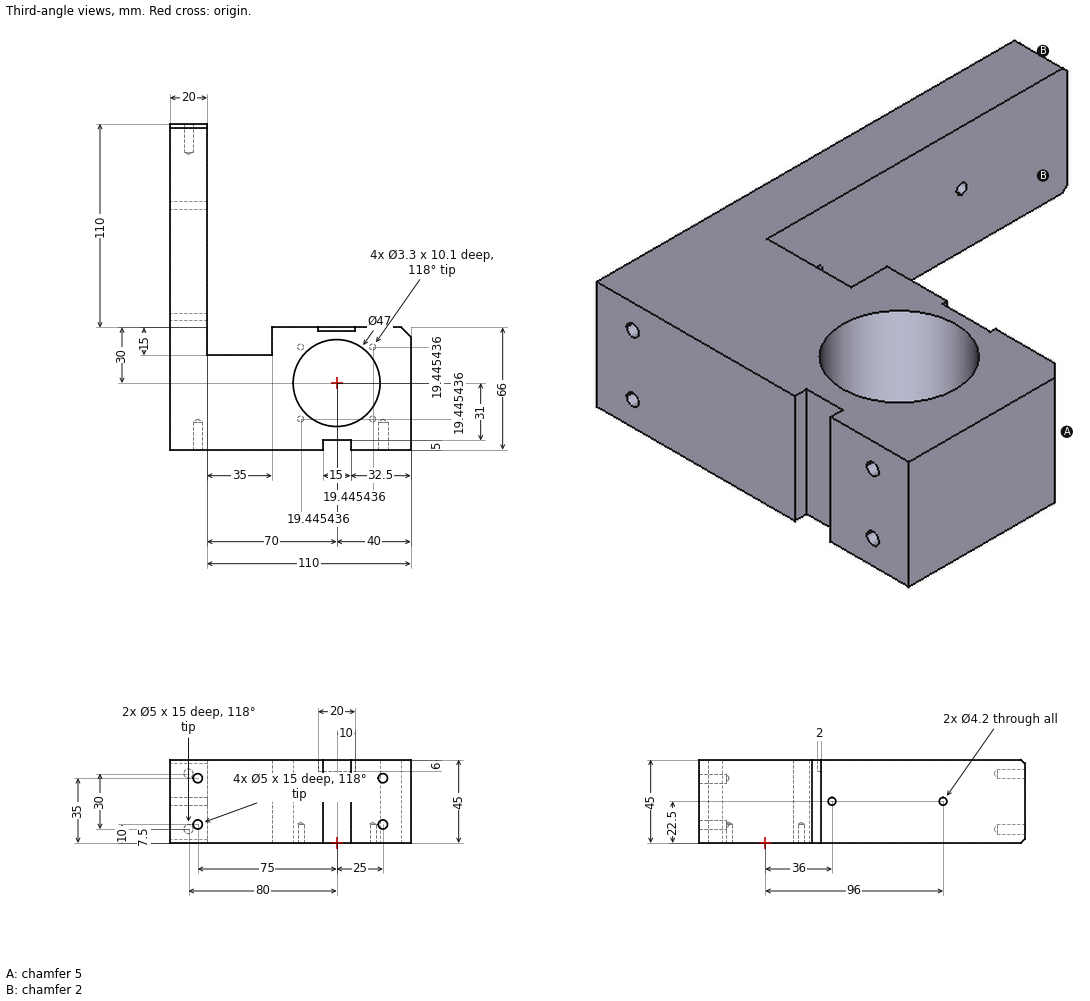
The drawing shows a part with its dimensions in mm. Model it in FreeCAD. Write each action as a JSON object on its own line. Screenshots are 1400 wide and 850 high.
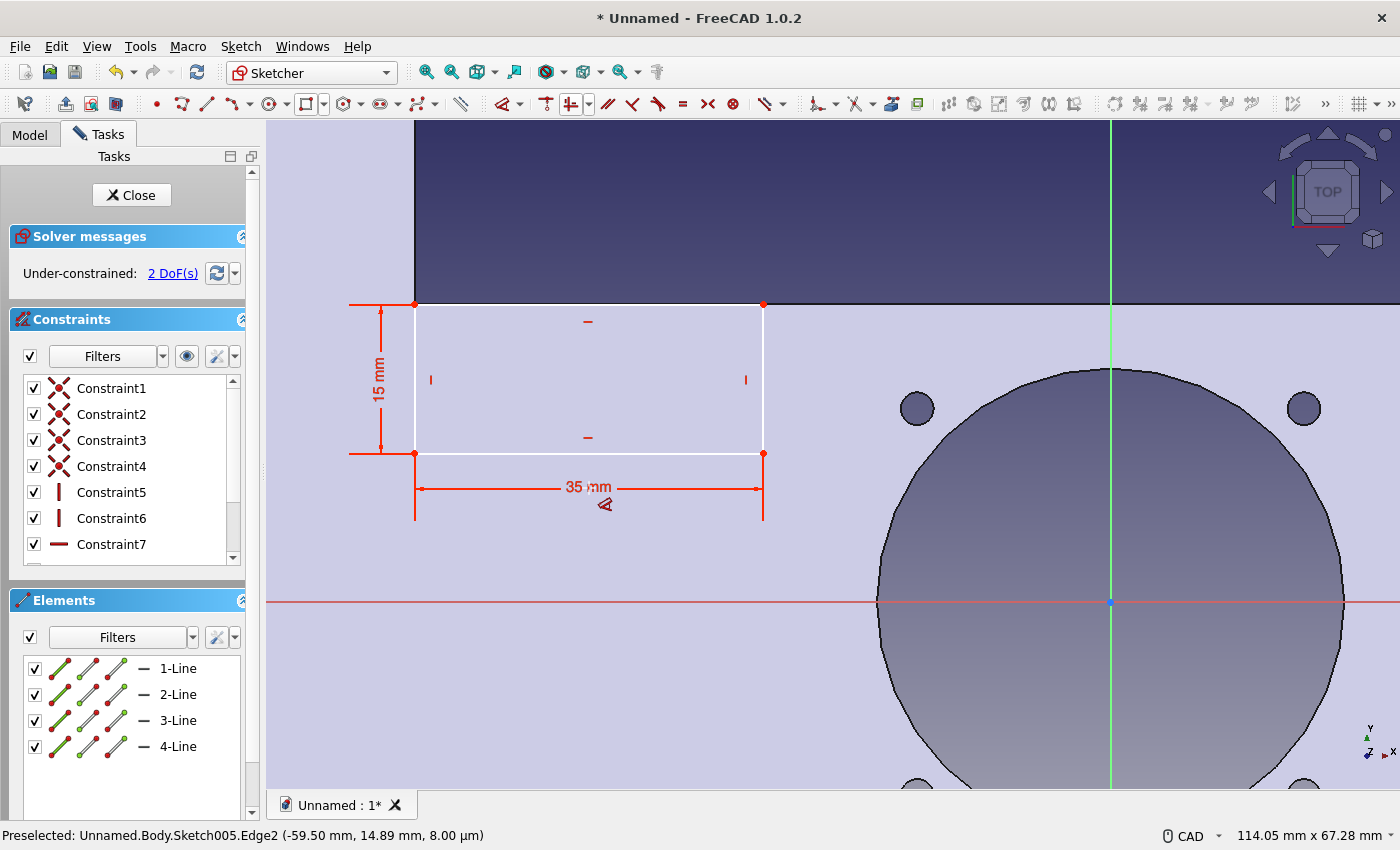
{"action": "left_click", "coordinate": [415, 305]}
{"action": "left_click", "coordinate": [763, 636]}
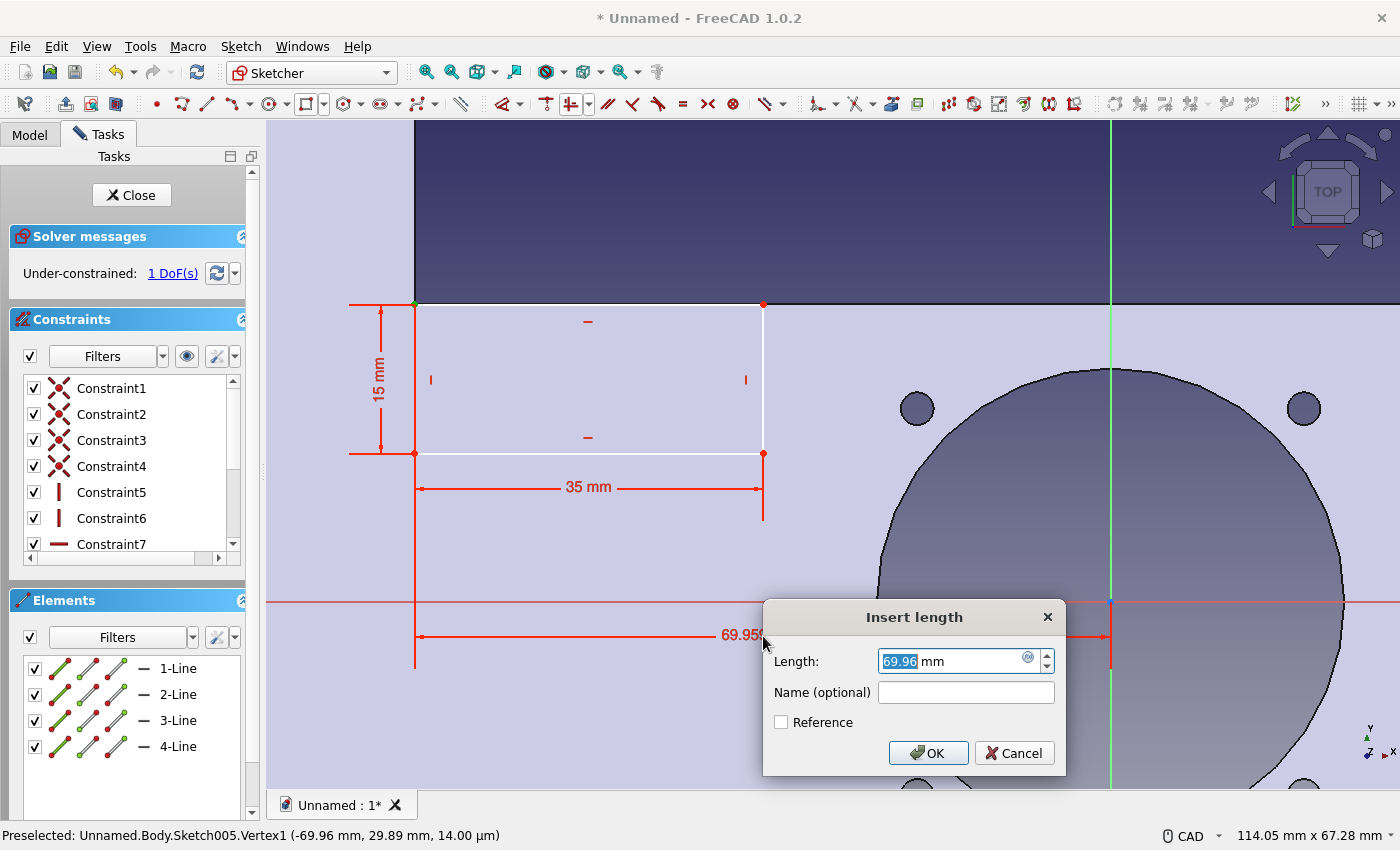
{"action": "type", "text": "70"}
{"action": "key", "text": "Return"}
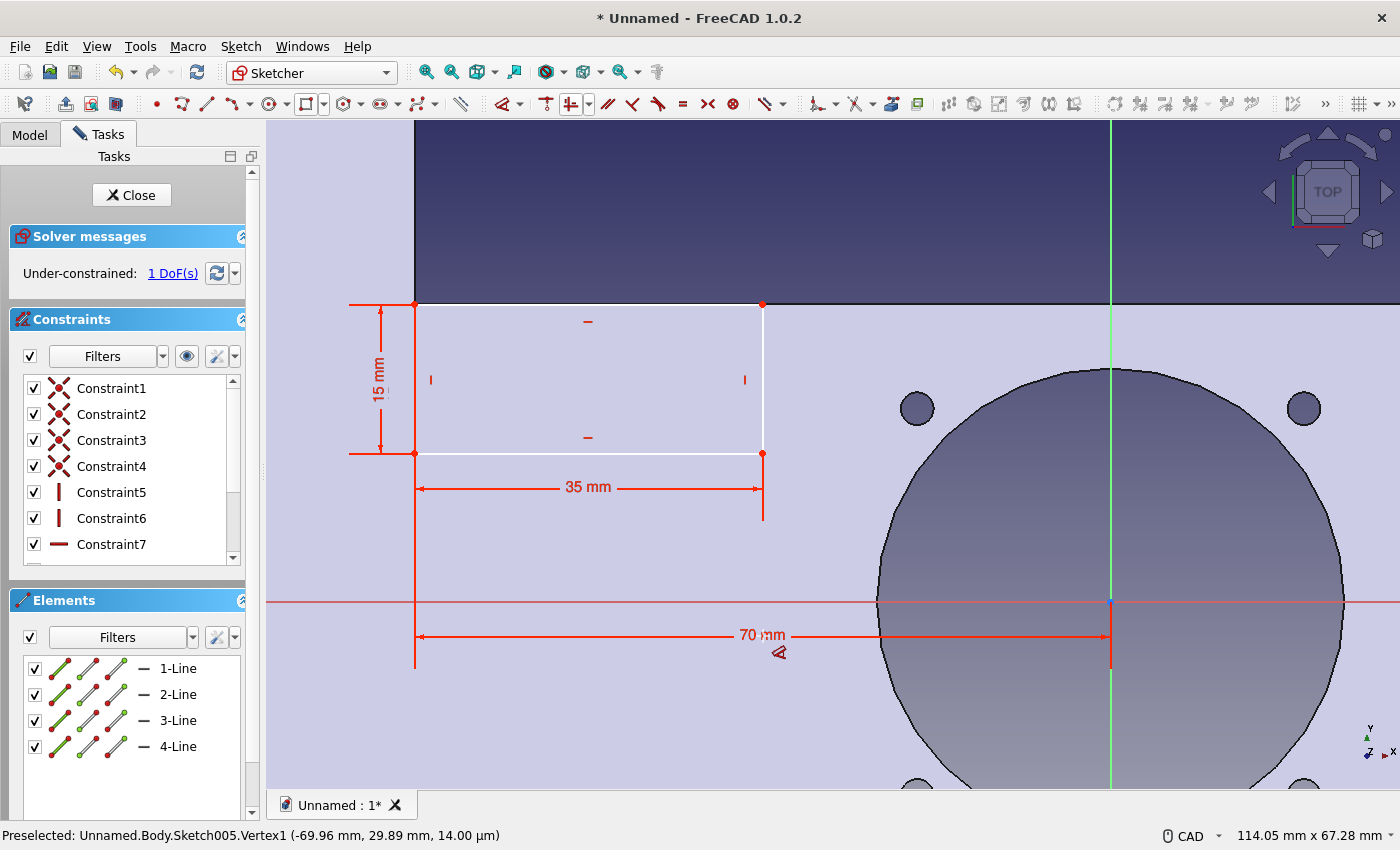
{"action": "left_click", "coordinate": [415, 305]}
{"action": "left_click", "coordinate": [1145, 453]}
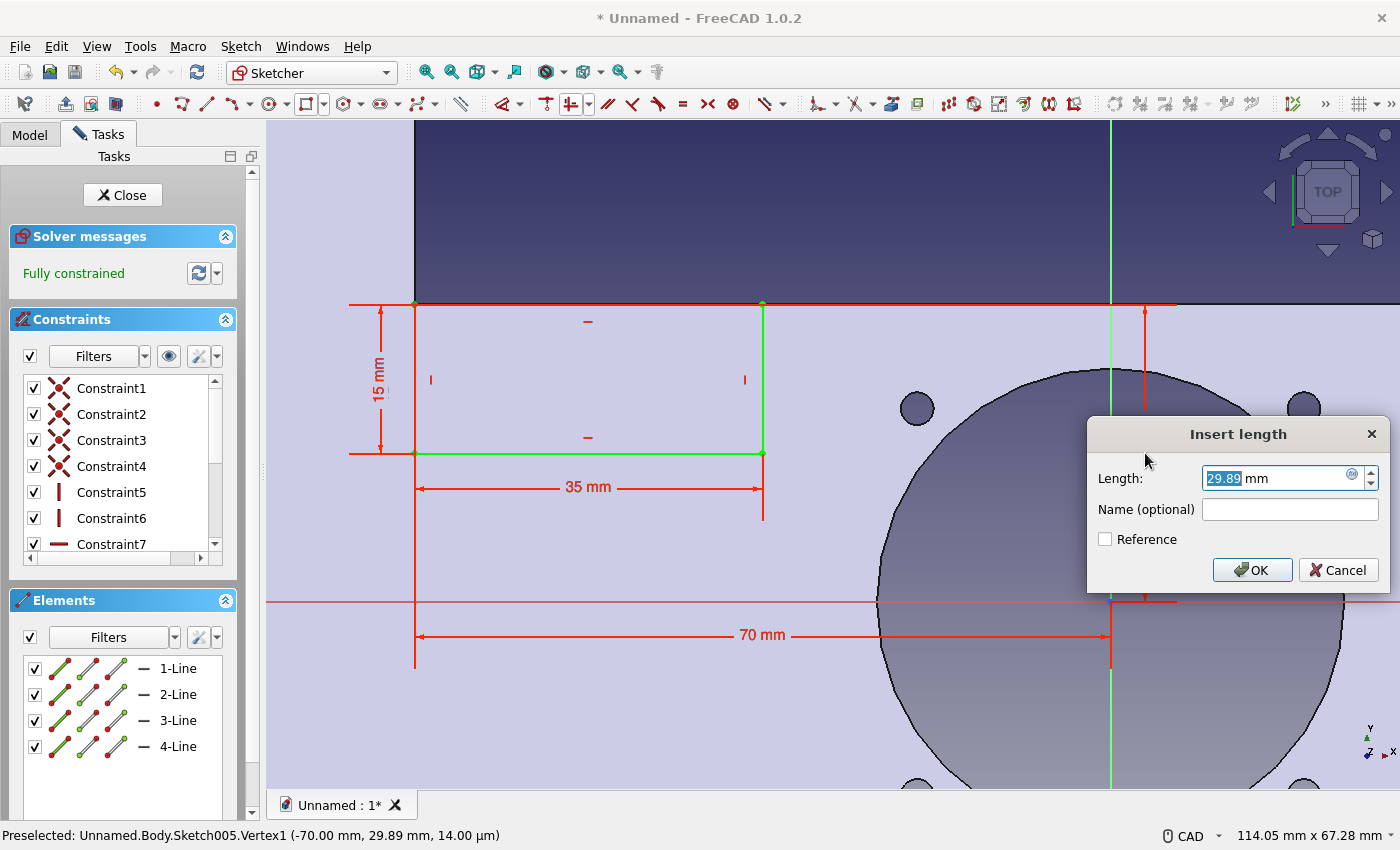
{"action": "type", "text": "30"}
{"action": "key", "text": "Return"}
{"action": "key", "text": "Escape"}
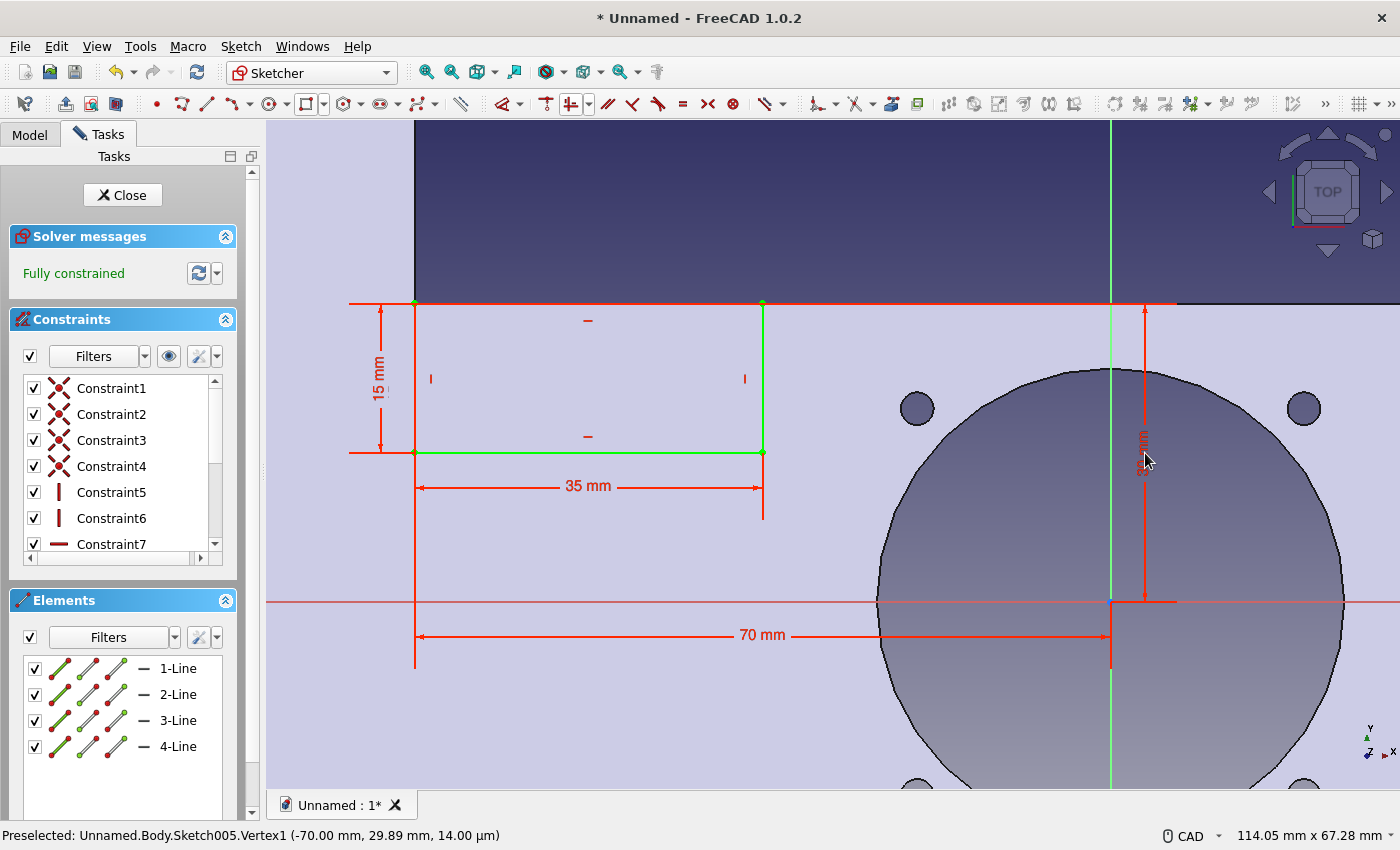
{"action": "left_click", "coordinate": [123, 195]}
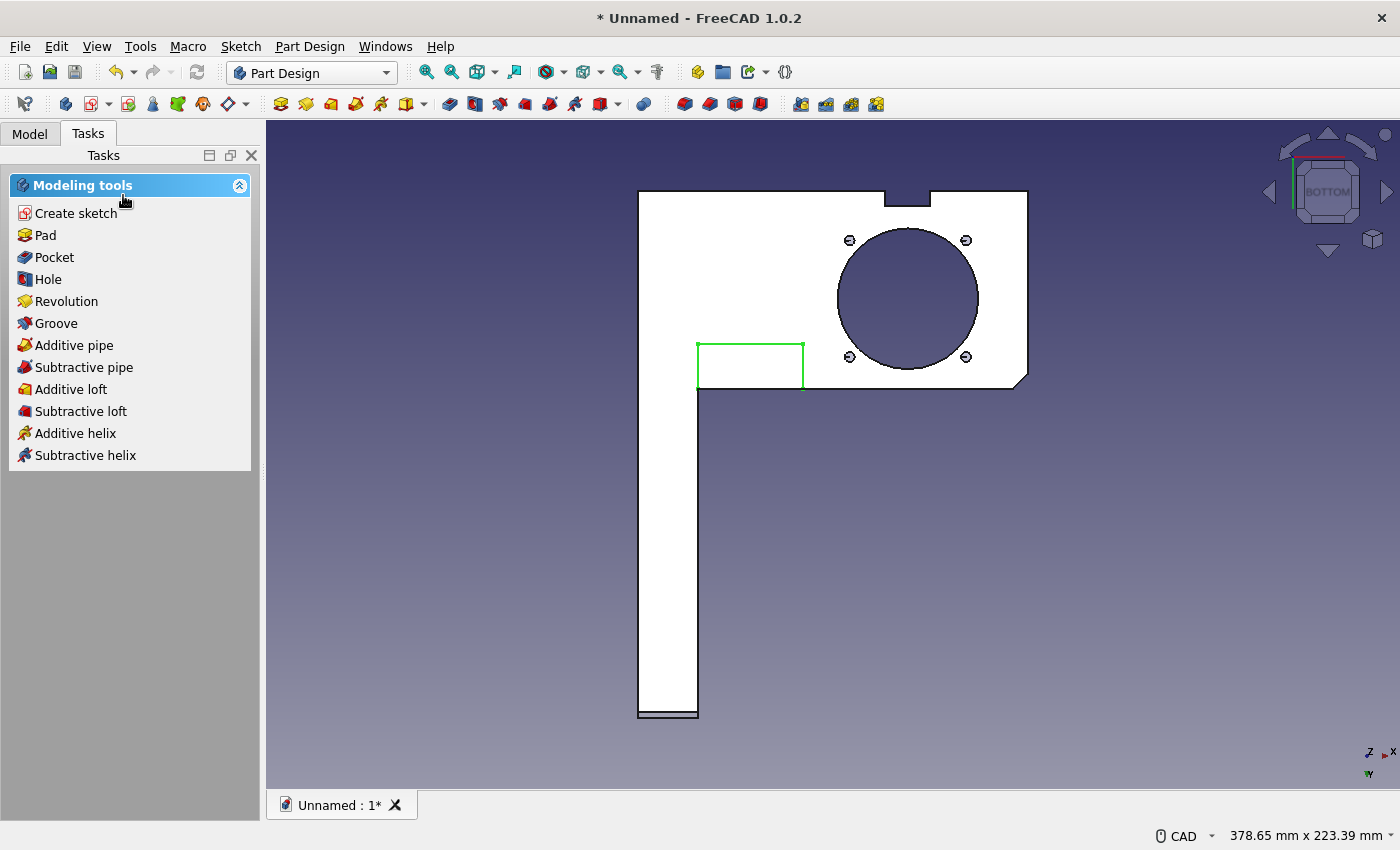
{"action": "left_click", "coordinate": [450, 104]}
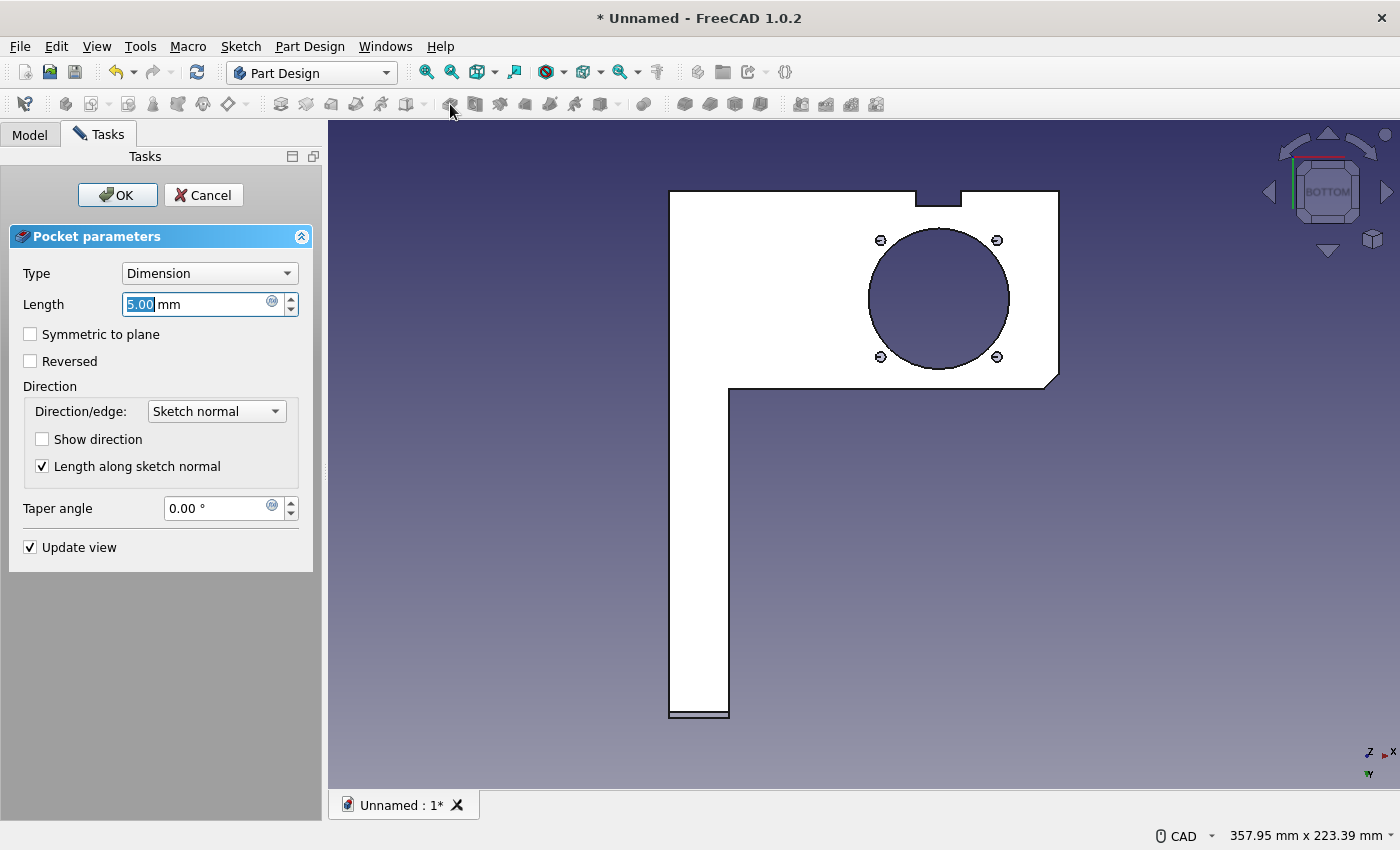
{"action": "left_click", "coordinate": [210, 274]}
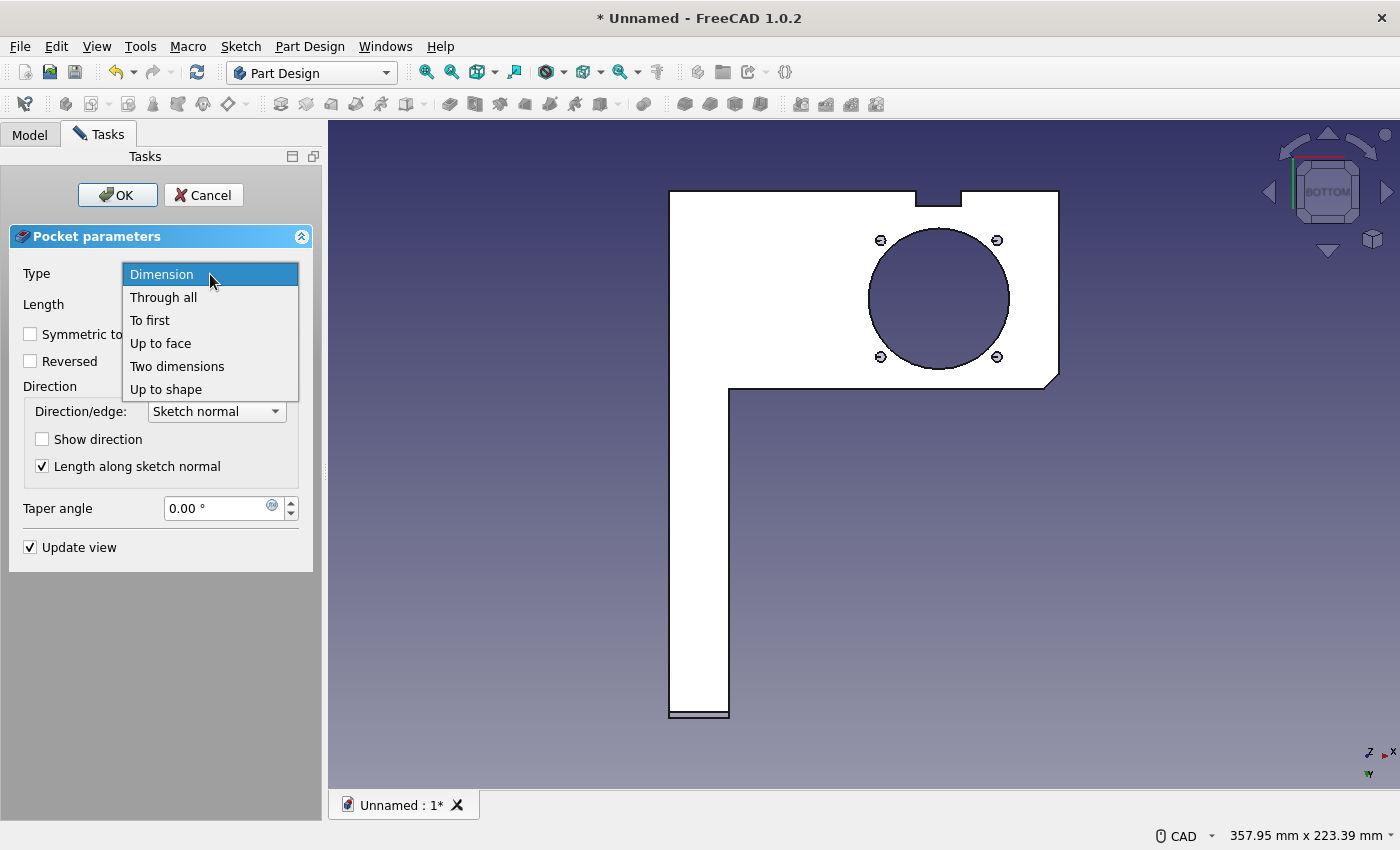
{"action": "left_click", "coordinate": [208, 298]}